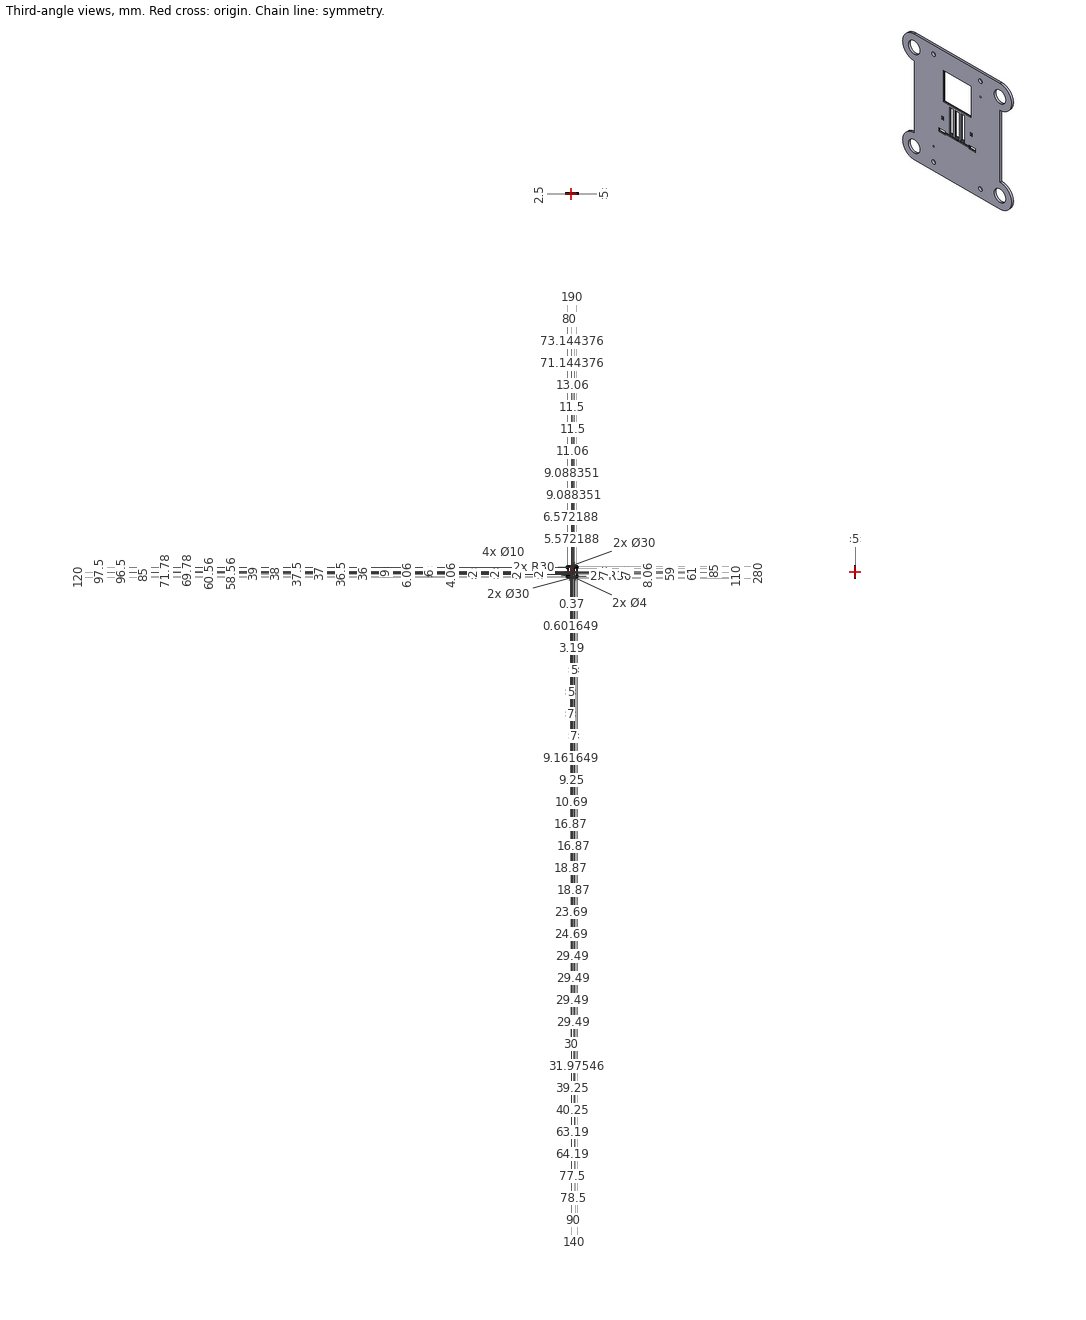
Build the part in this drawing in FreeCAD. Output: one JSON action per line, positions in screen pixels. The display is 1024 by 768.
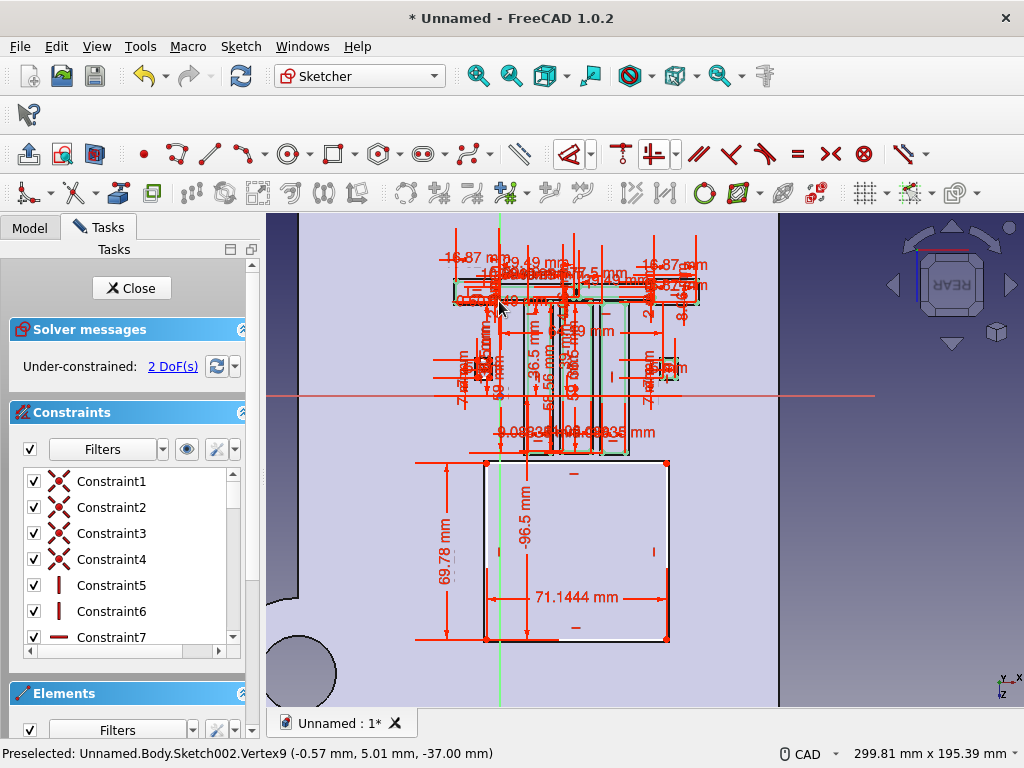
{"action": "scroll", "coordinate": [487, 463], "scroll_direction": "up", "scroll_amount": 6}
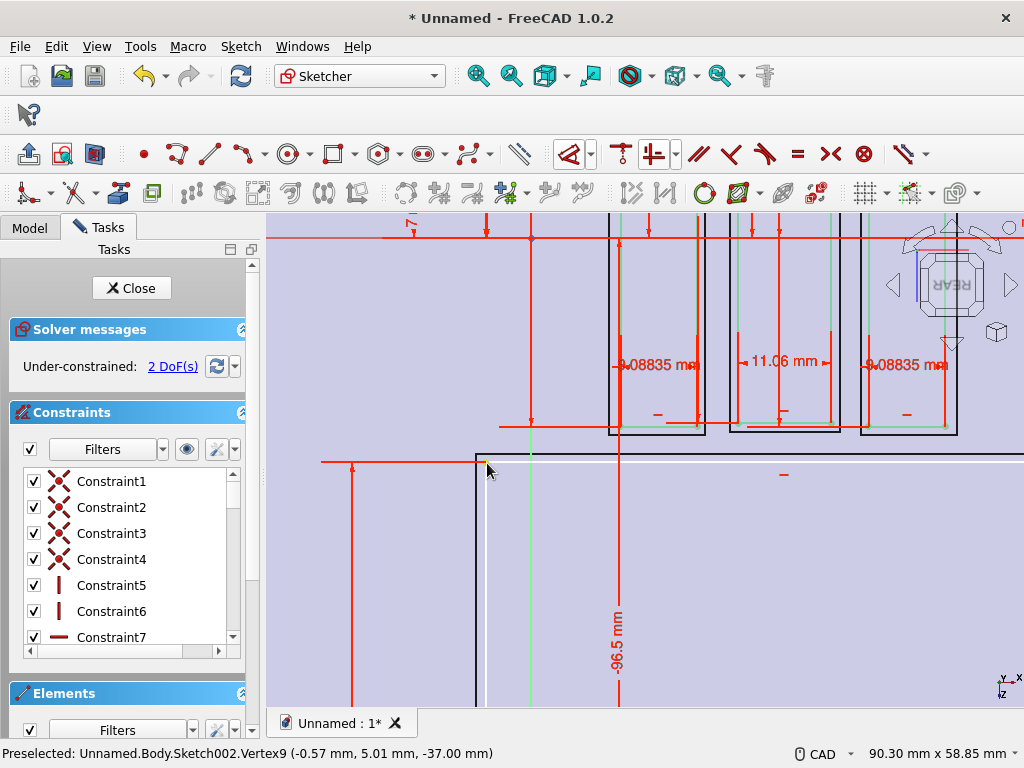
{"action": "left_click", "coordinate": [486, 462]}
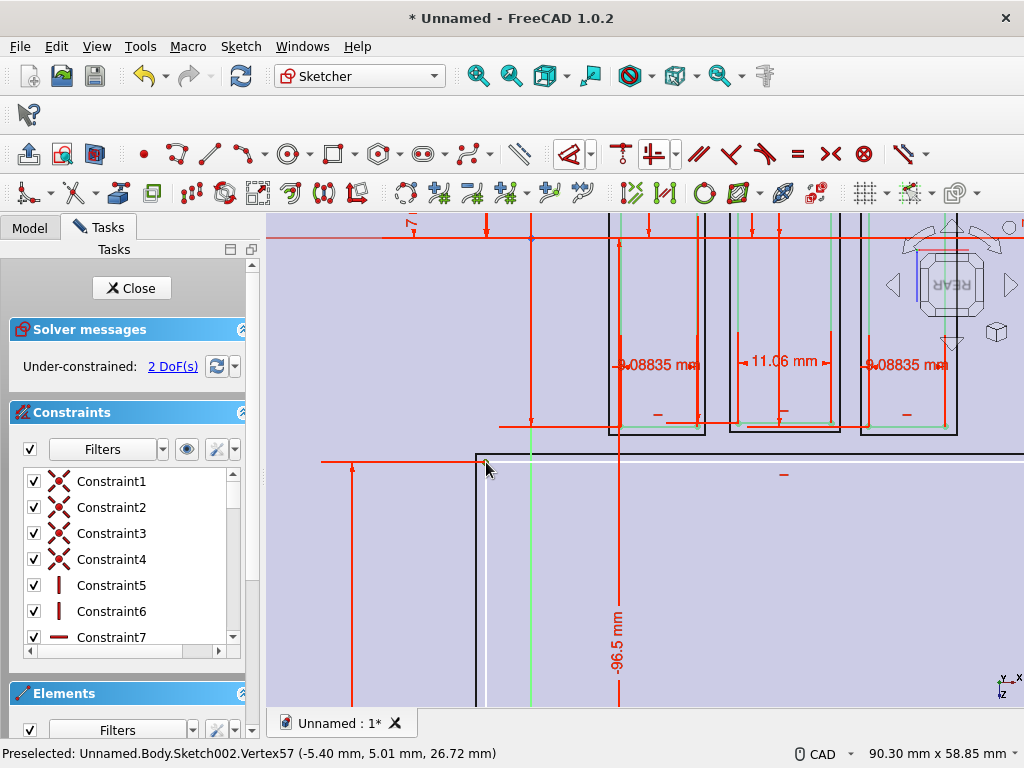
{"action": "key", "text": "l"}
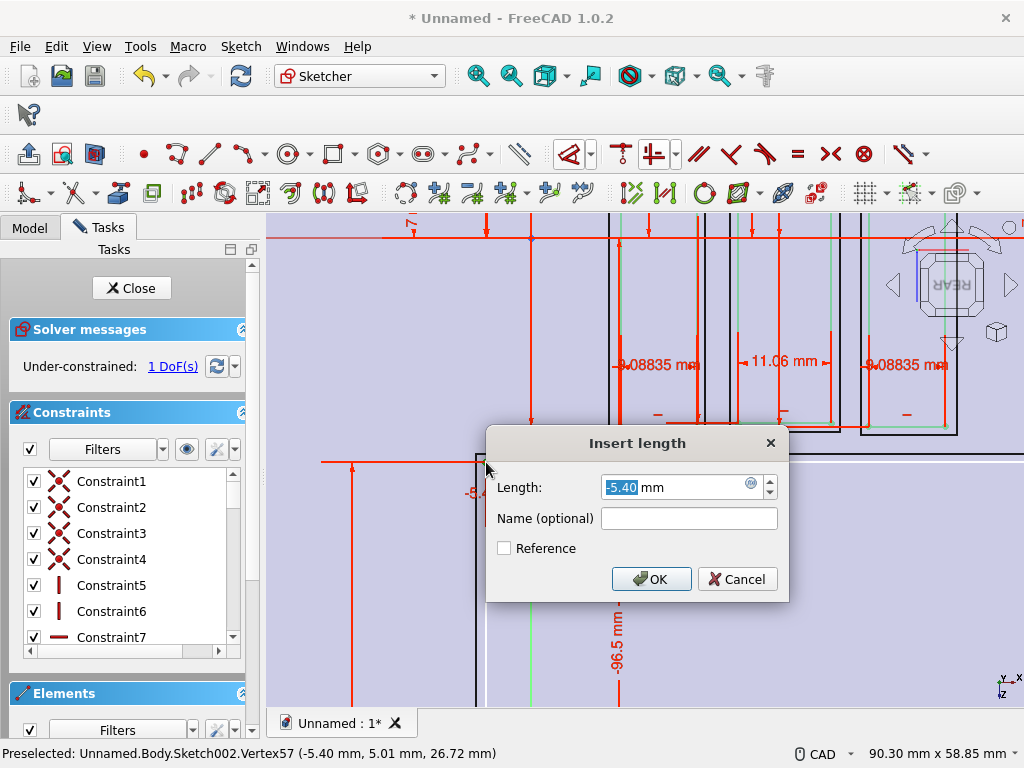
{"action": "type", "text": "-5.572188"}
{"action": "key", "text": "Return"}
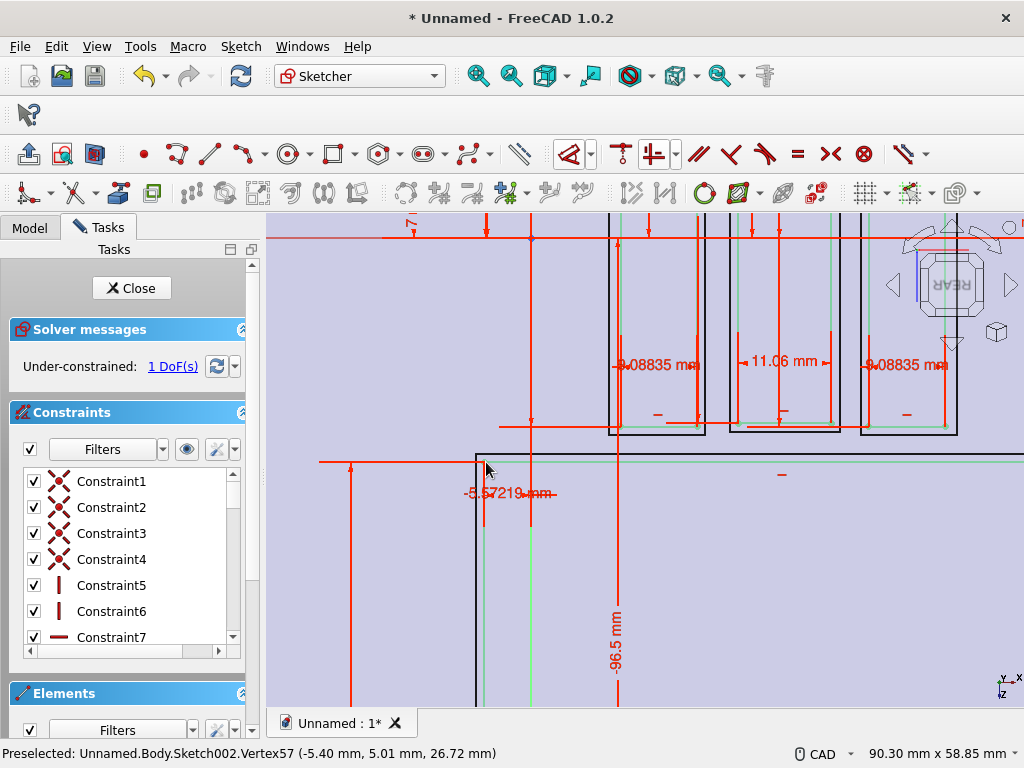
{"action": "scroll", "coordinate": [509, 462], "scroll_direction": "down", "scroll_amount": 7}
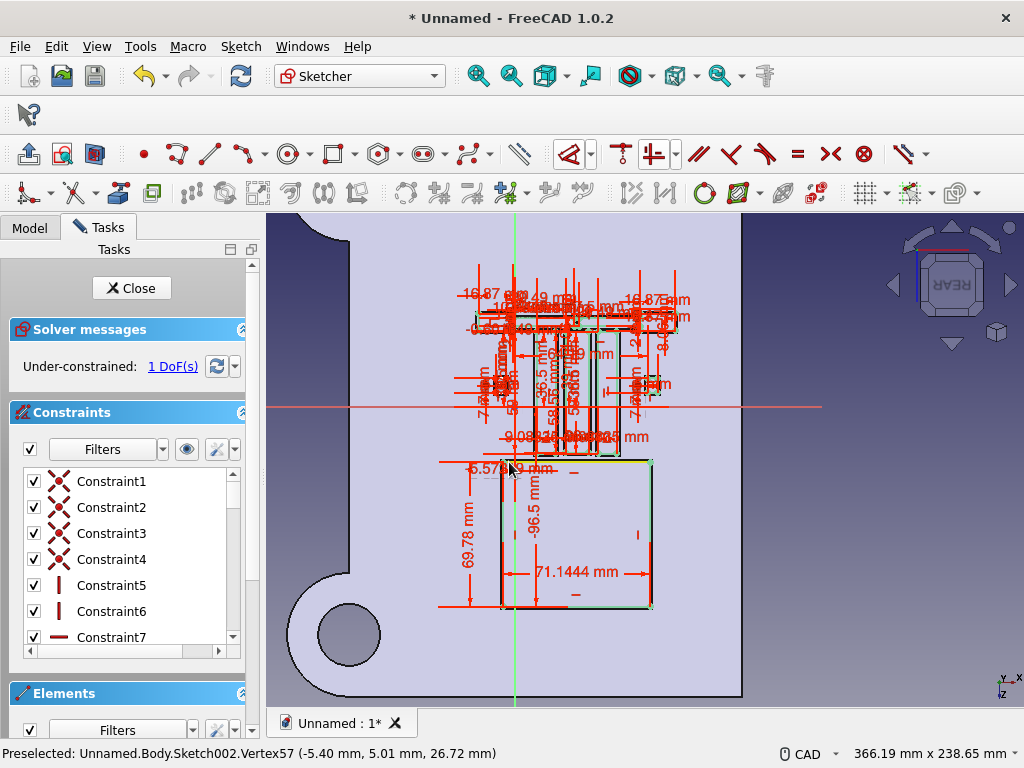
{"action": "scroll", "coordinate": [496, 378], "scroll_direction": "up", "scroll_amount": 4}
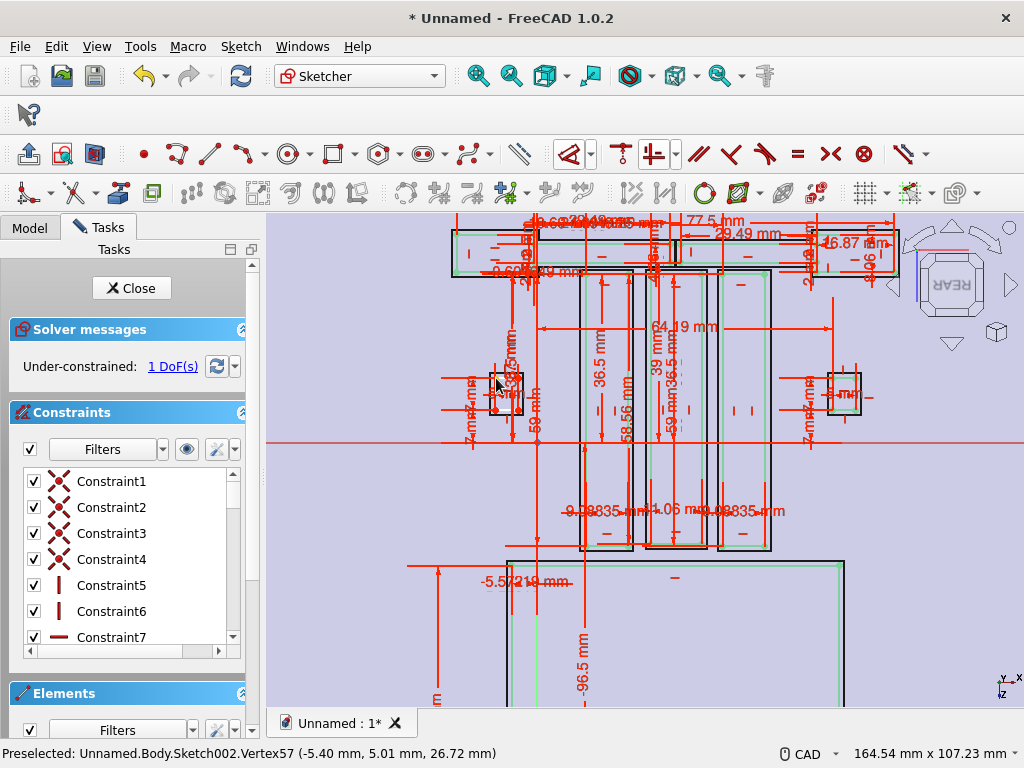
{"action": "left_click", "coordinate": [495, 378]}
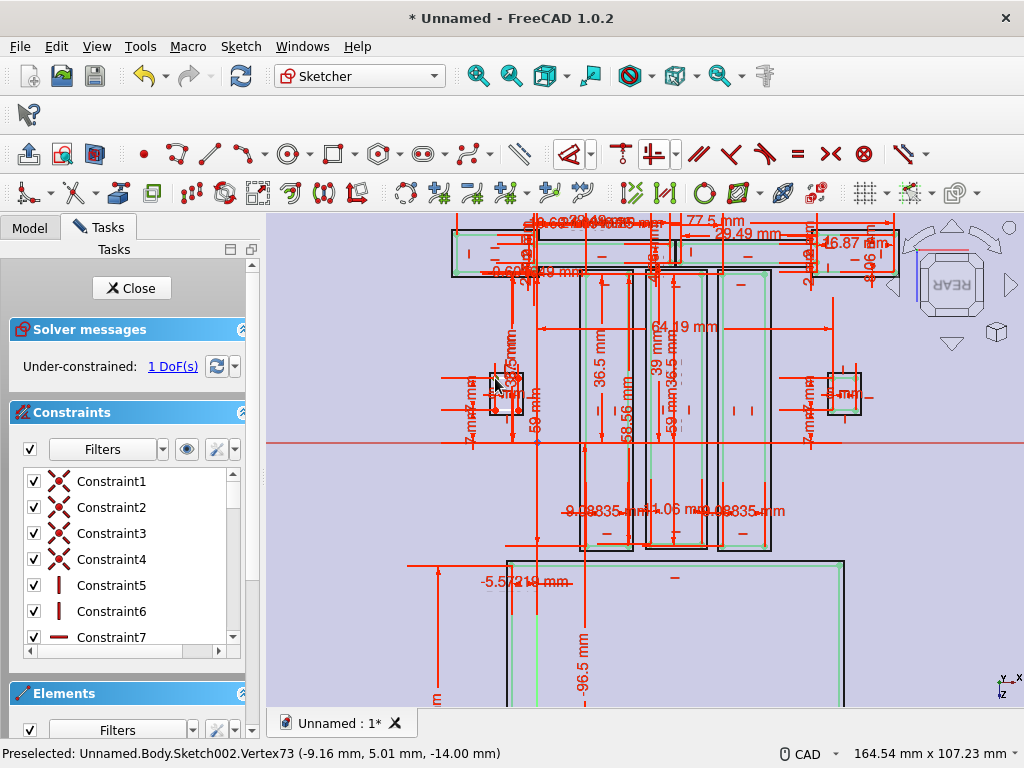
{"action": "key", "text": "l"}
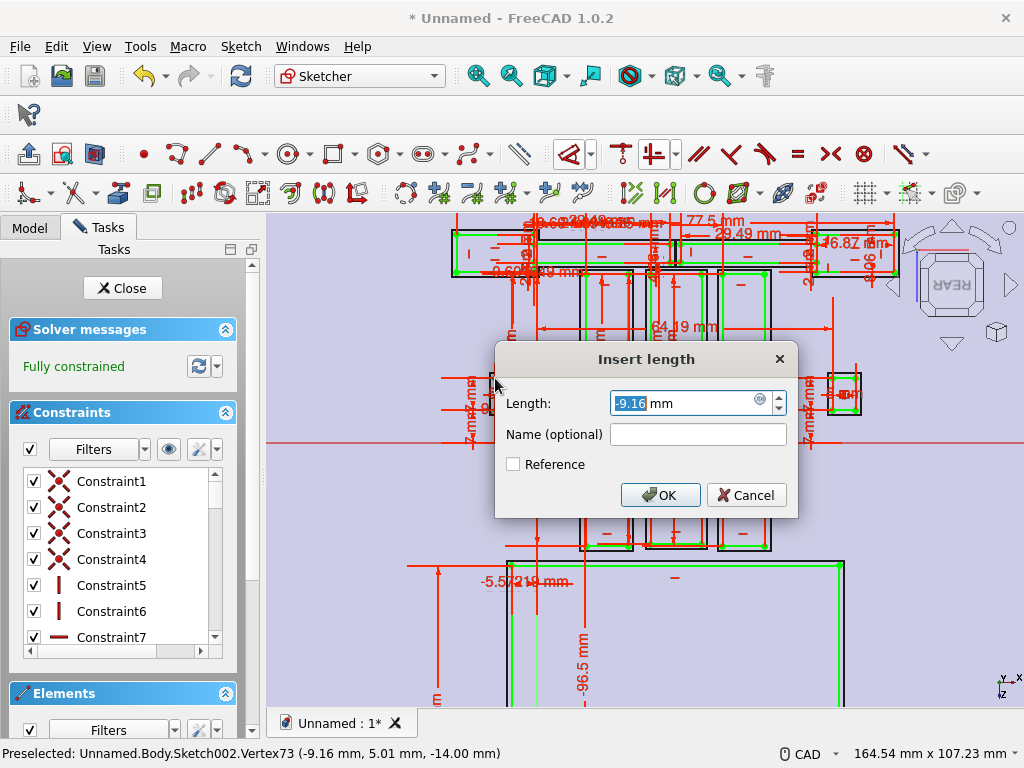
{"action": "type", "text": "-9.161649"}
{"action": "key", "text": "Return"}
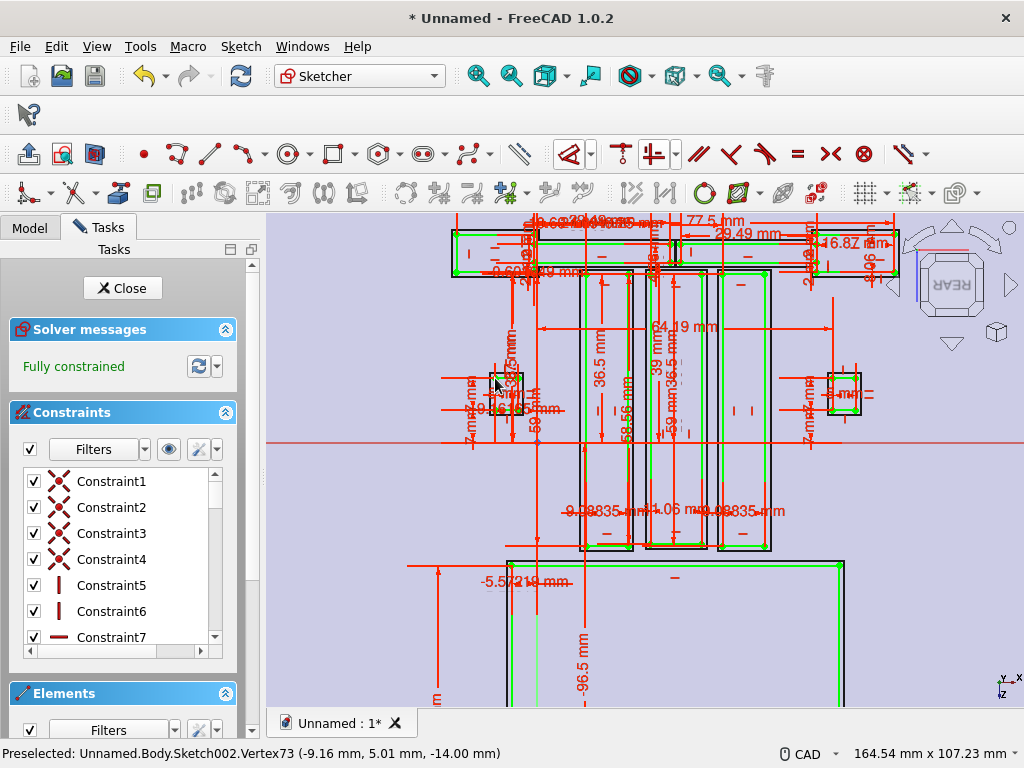
{"action": "left_click", "coordinate": [123, 288]}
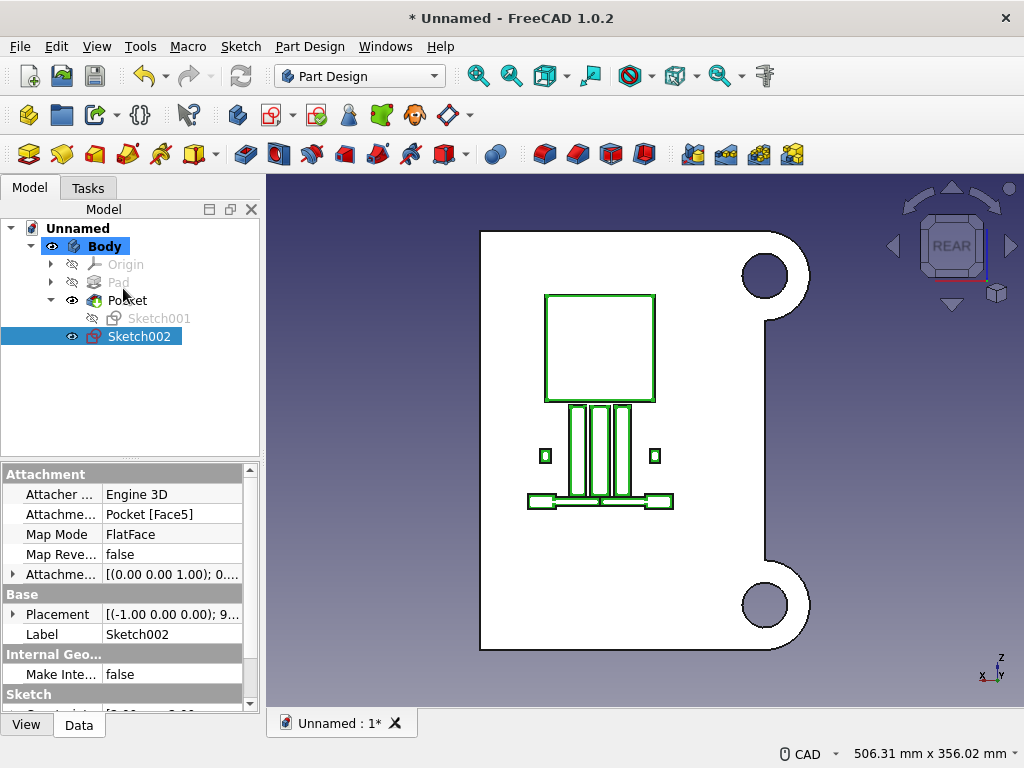
{"action": "left_click", "coordinate": [246, 154]}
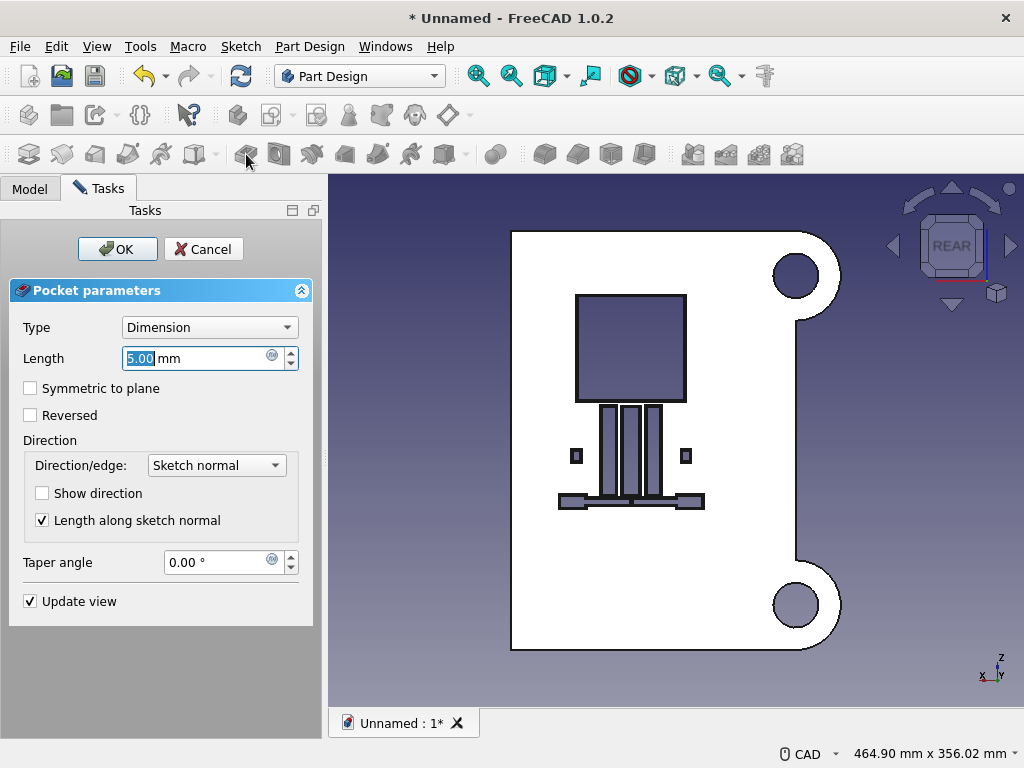
{"action": "type", "text": "5"}
{"action": "key", "text": "Tab"}